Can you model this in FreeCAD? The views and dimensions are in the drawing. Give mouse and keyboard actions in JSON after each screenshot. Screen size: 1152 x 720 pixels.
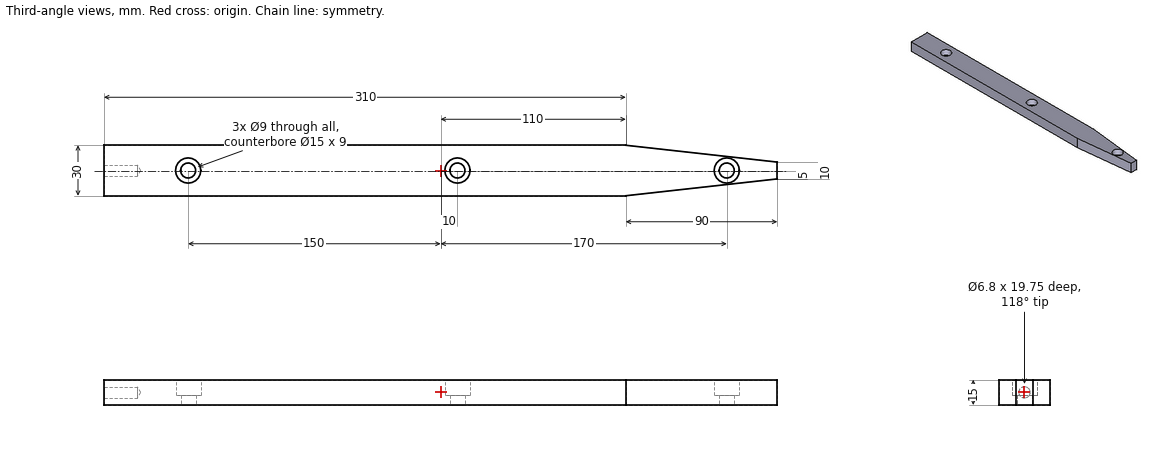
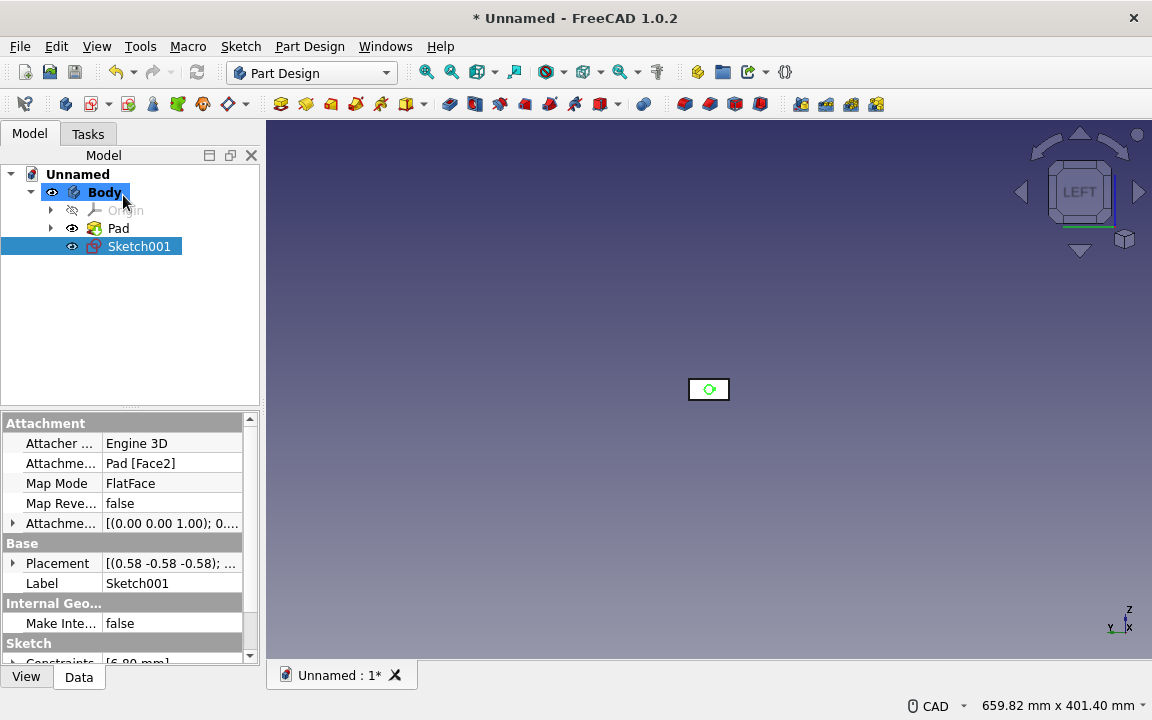
{"action": "left_click", "coordinate": [475, 104]}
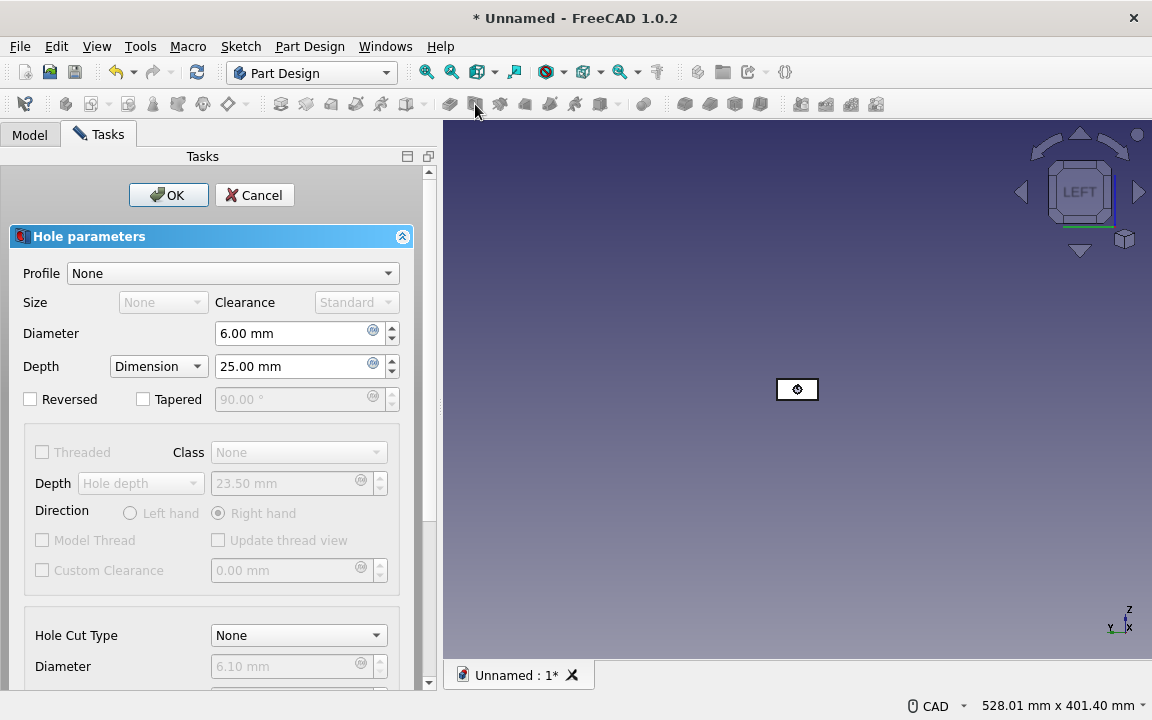
{"action": "triple_click", "coordinate": [300, 334]}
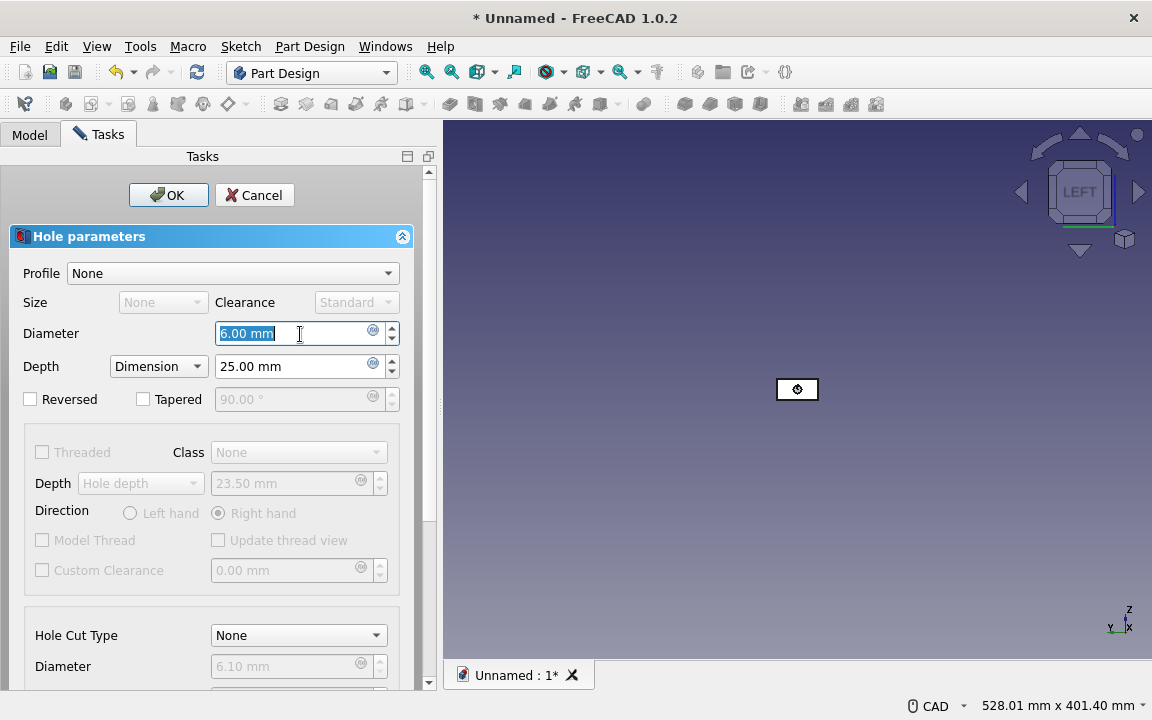
{"action": "type", "text": "6.8"}
{"action": "key", "text": "Tab"}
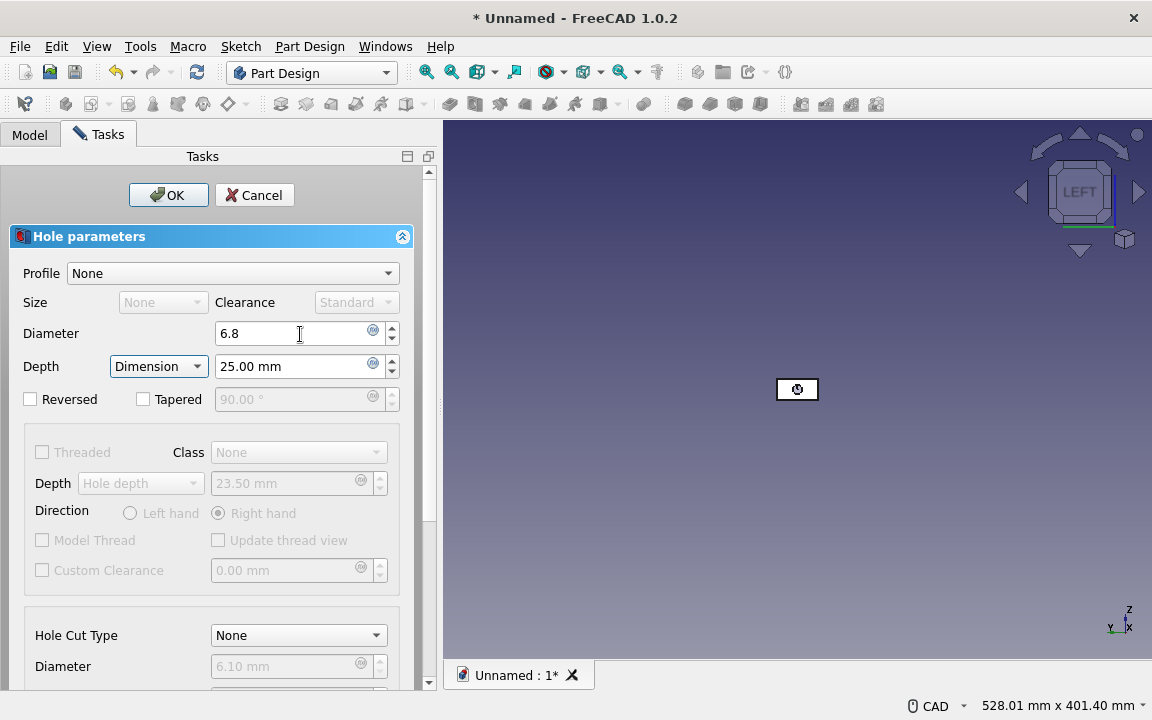
{"action": "triple_click", "coordinate": [300, 366]}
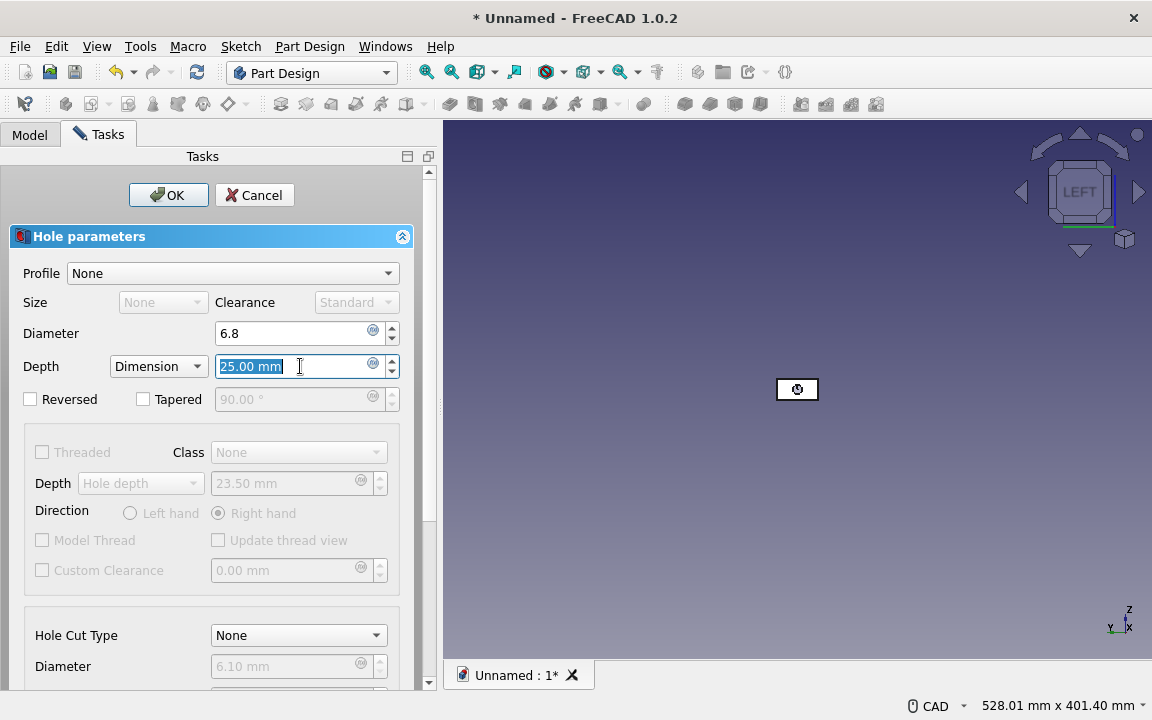
{"action": "type", "text": "19.75"}
{"action": "key", "text": "Tab"}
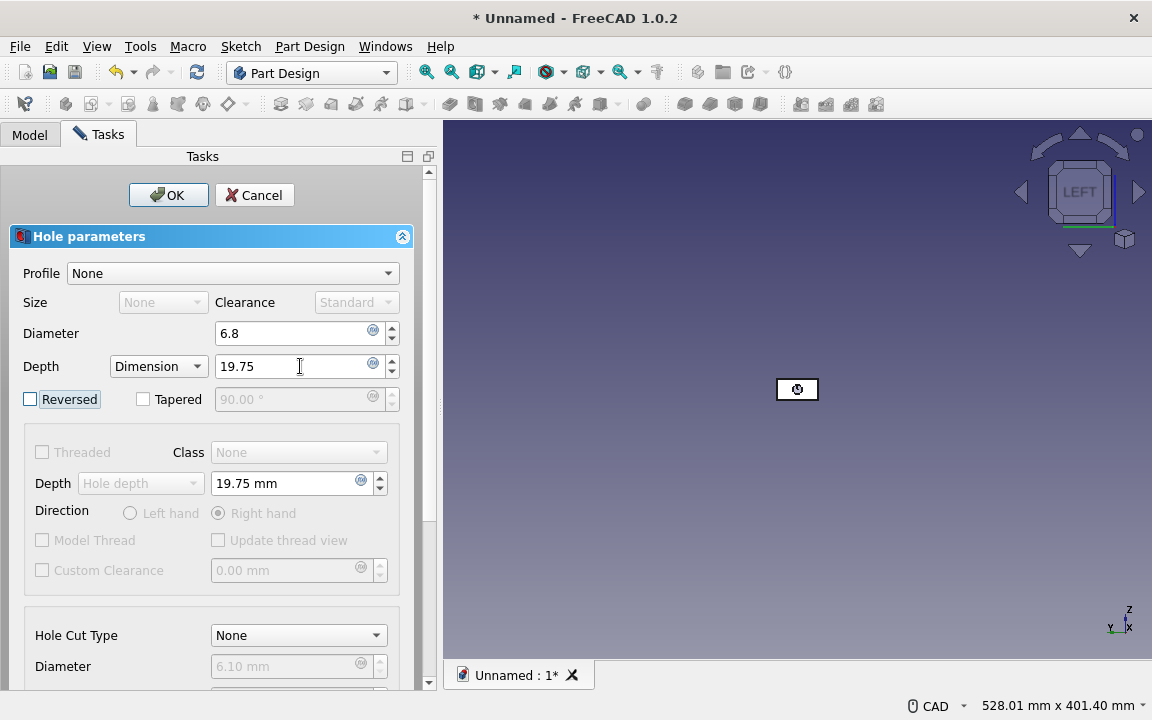
{"action": "left_click", "coordinate": [169, 195]}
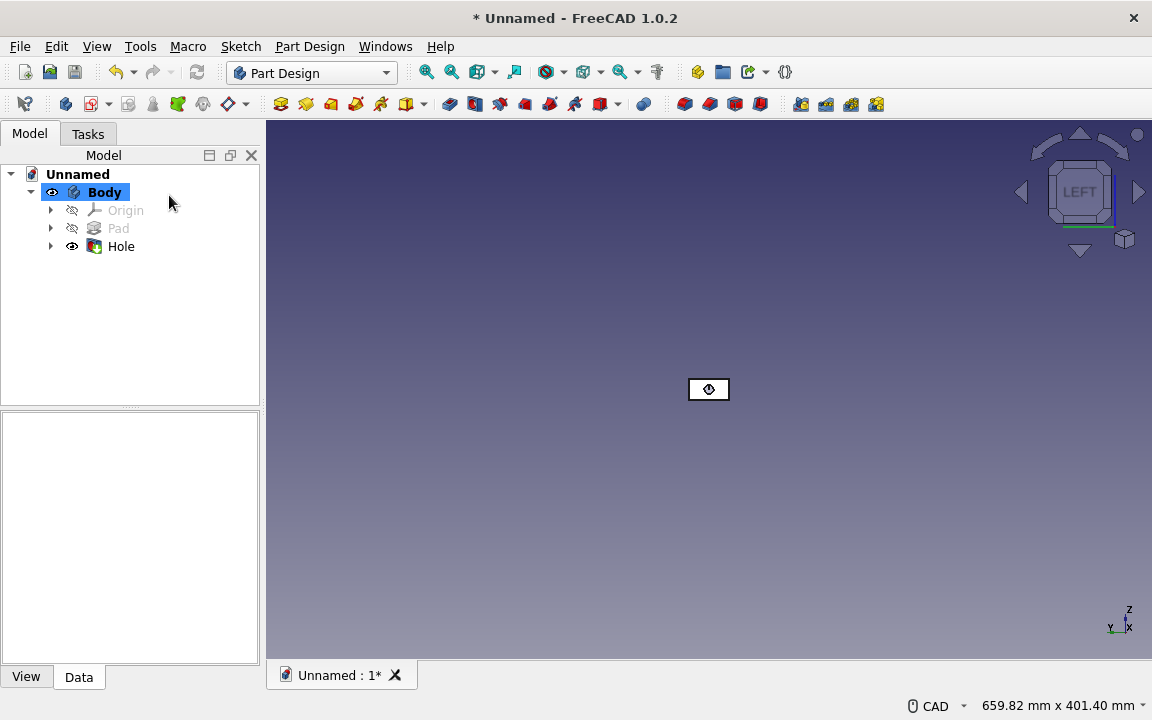
{"action": "key", "text": "v f"}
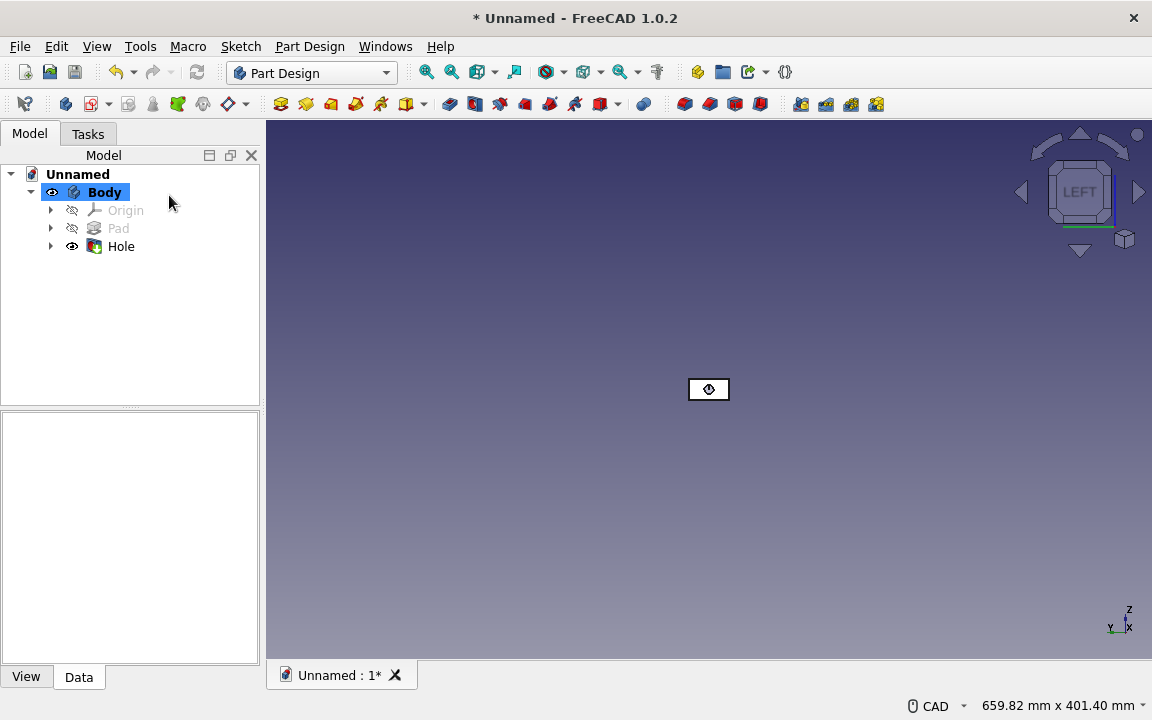
{"action": "key", "text": "0"}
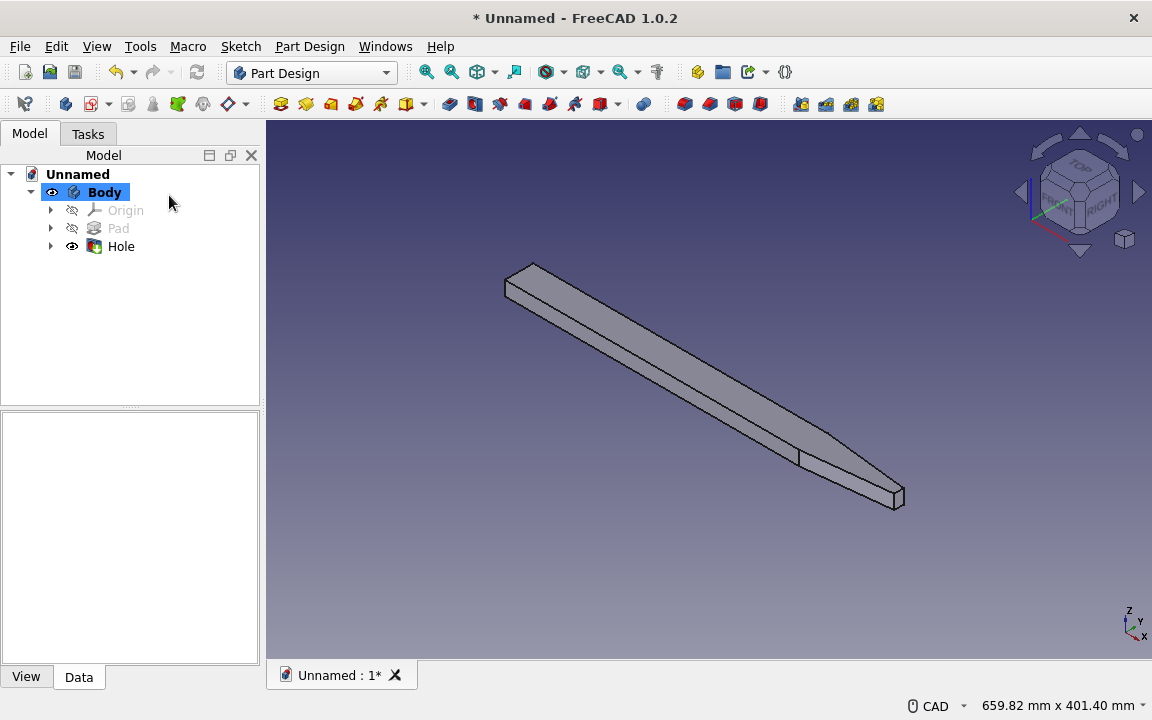
{"action": "left_click", "coordinate": [763, 412]}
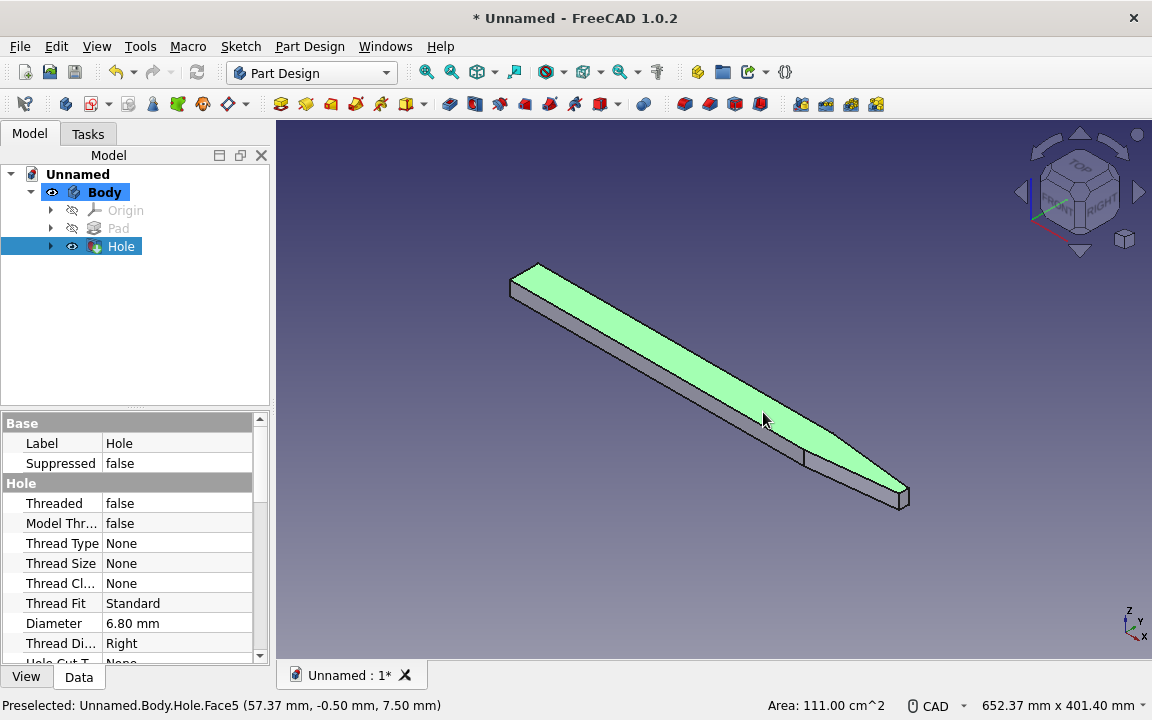
{"action": "left_click", "coordinate": [90, 104]}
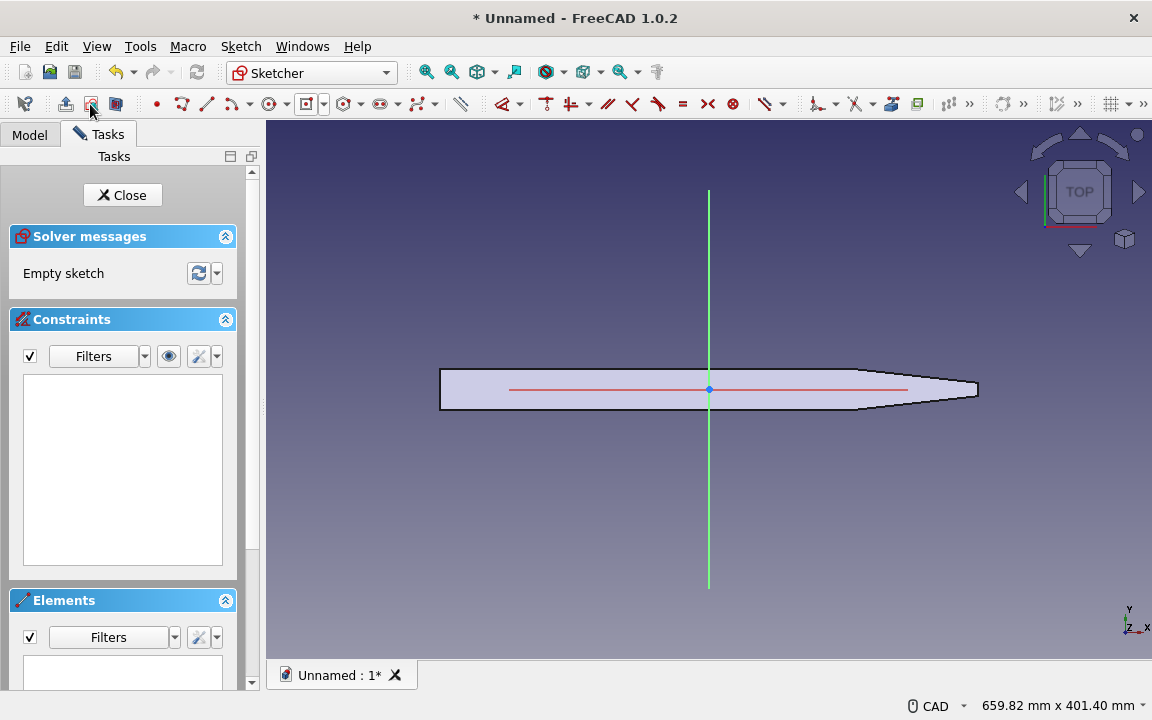
{"action": "left_click", "coordinate": [268, 104]}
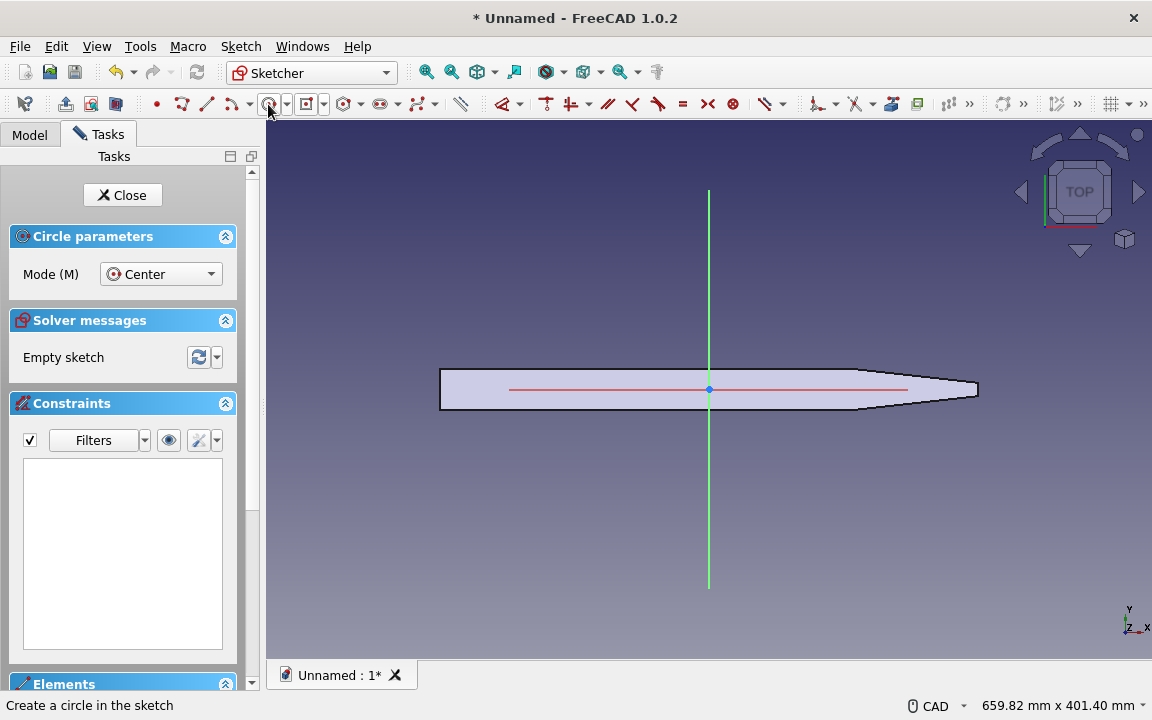
{"action": "scroll", "coordinate": [508, 390], "scroll_direction": "up", "scroll_amount": 7}